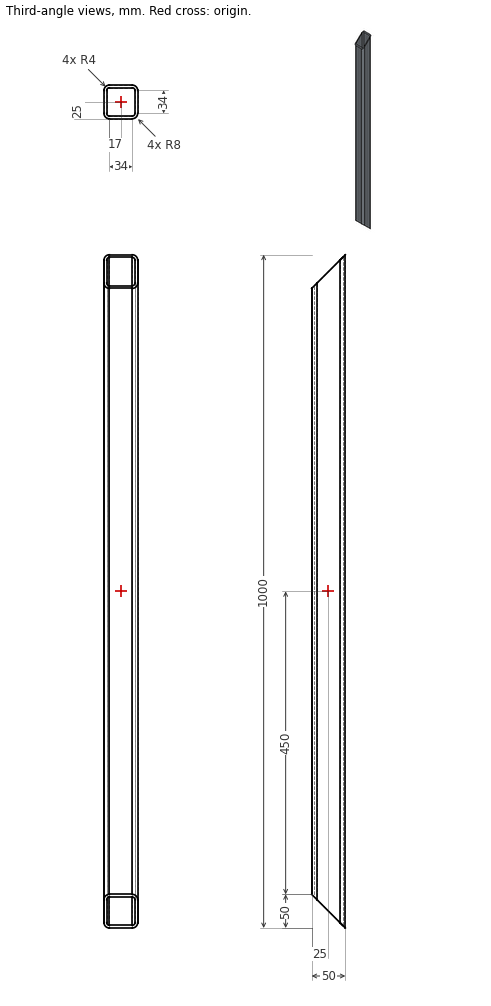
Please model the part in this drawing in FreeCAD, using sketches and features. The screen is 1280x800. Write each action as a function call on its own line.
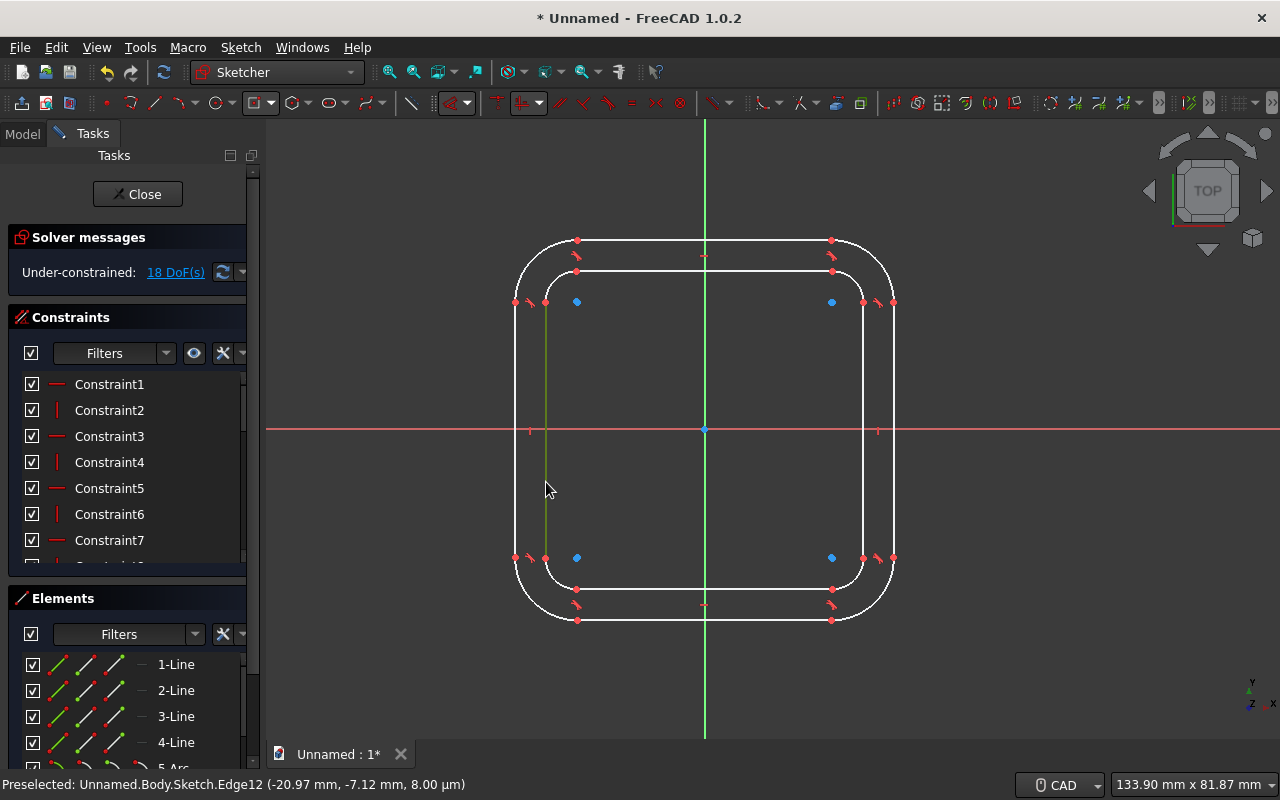
click(549, 572)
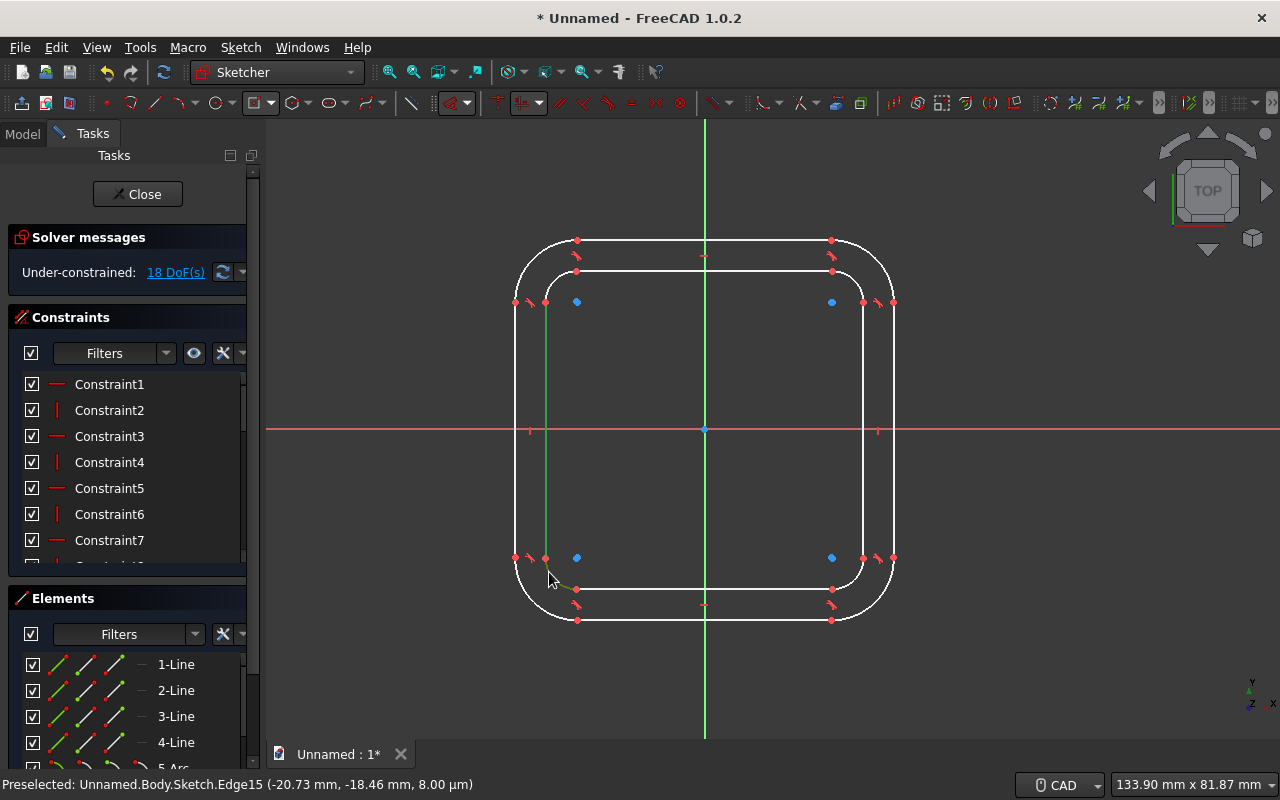
click(608, 104)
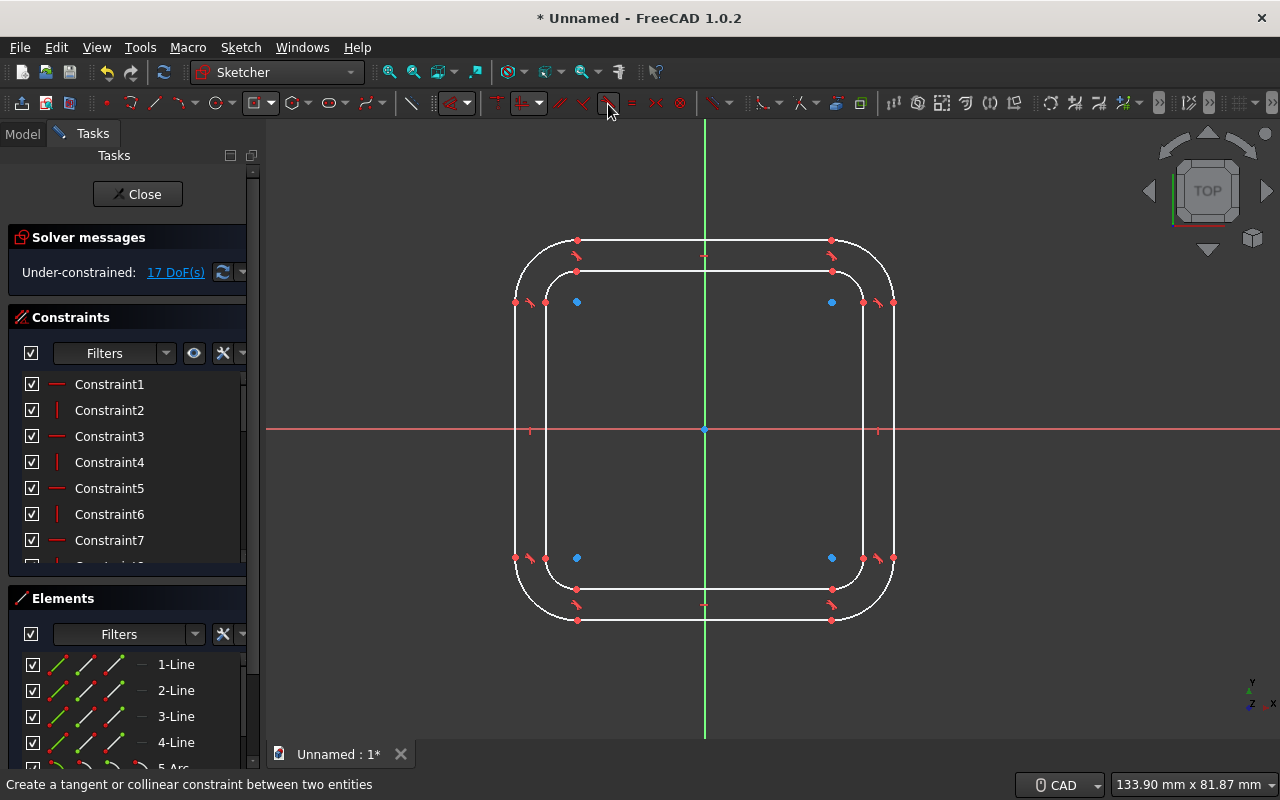
click(546, 482)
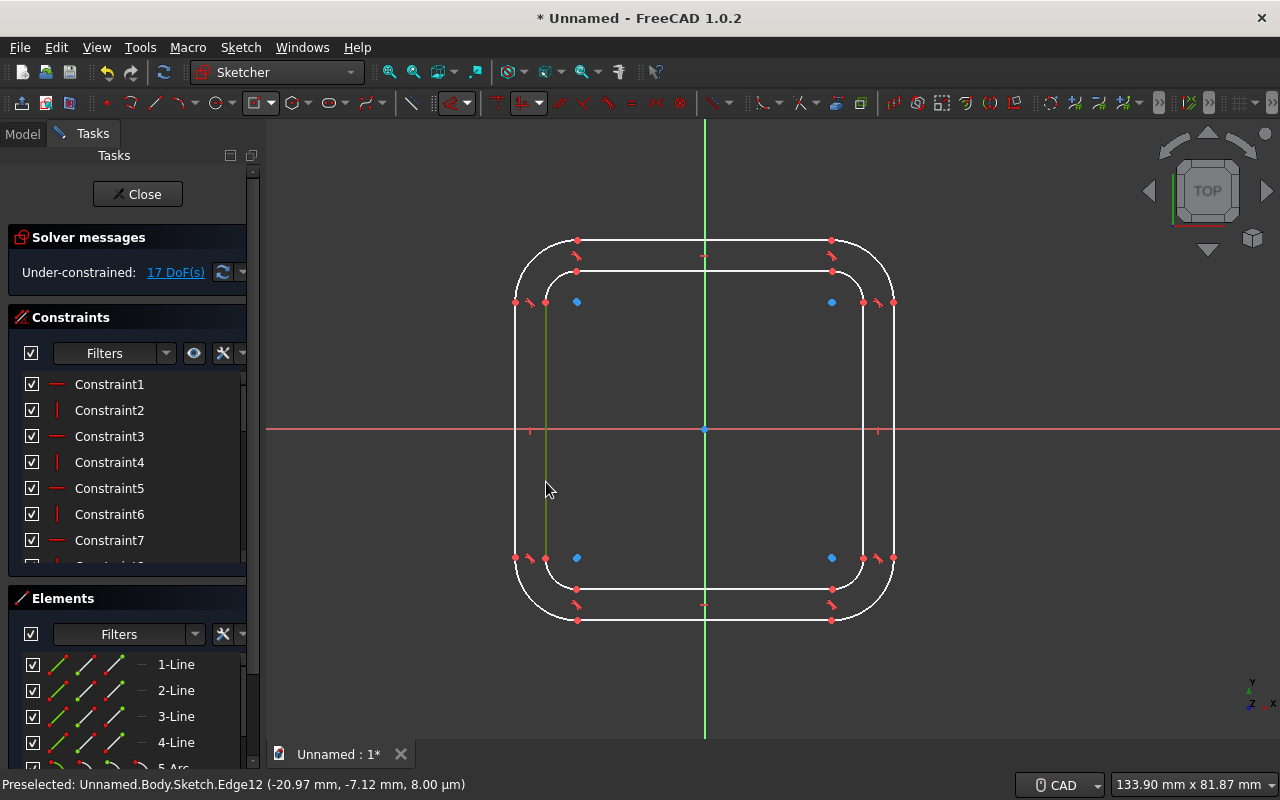
click(562, 275)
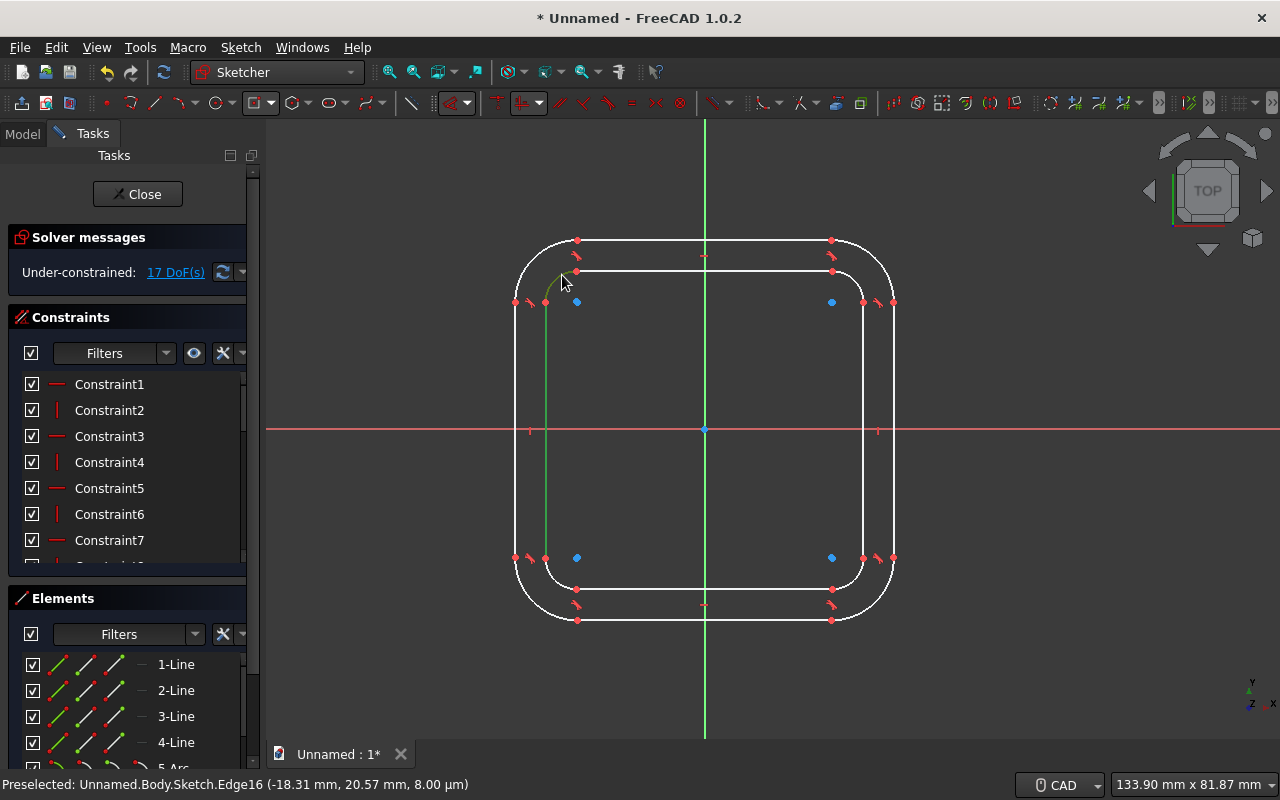
click(608, 104)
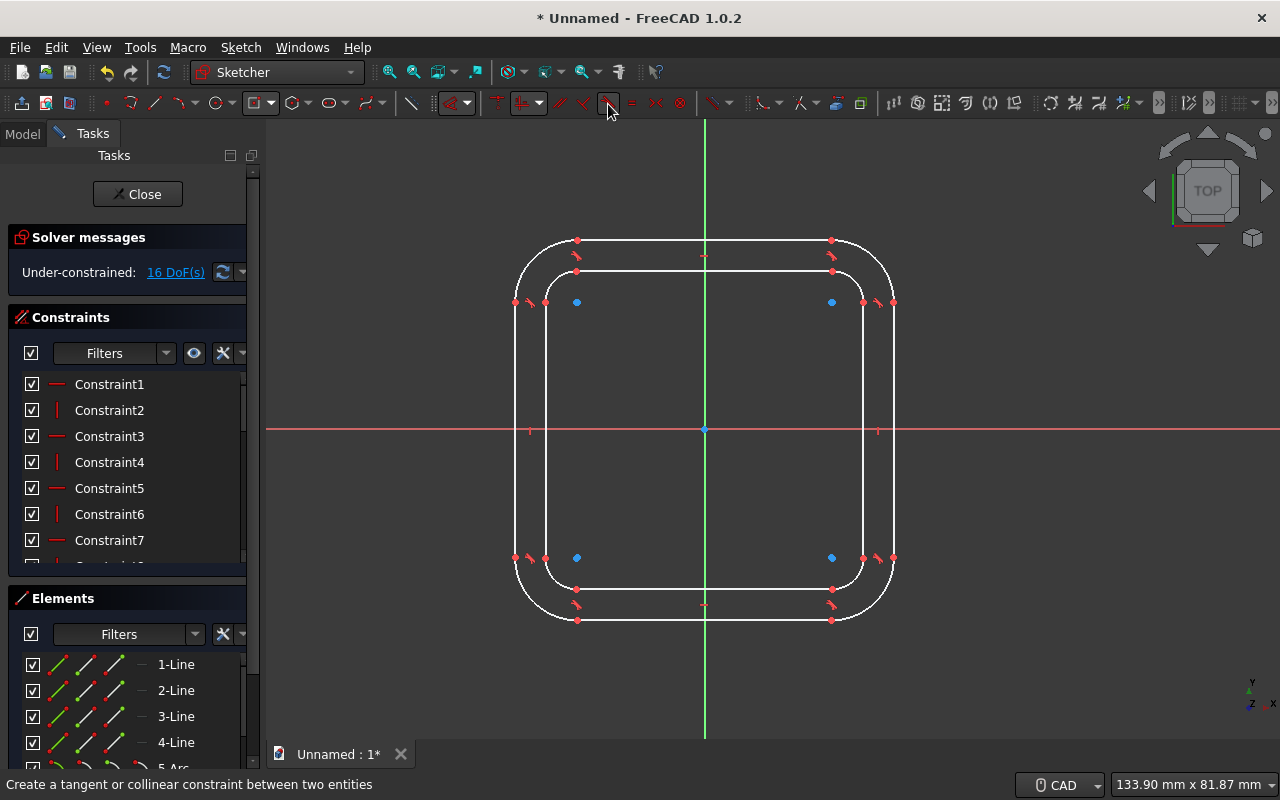
click(887, 274)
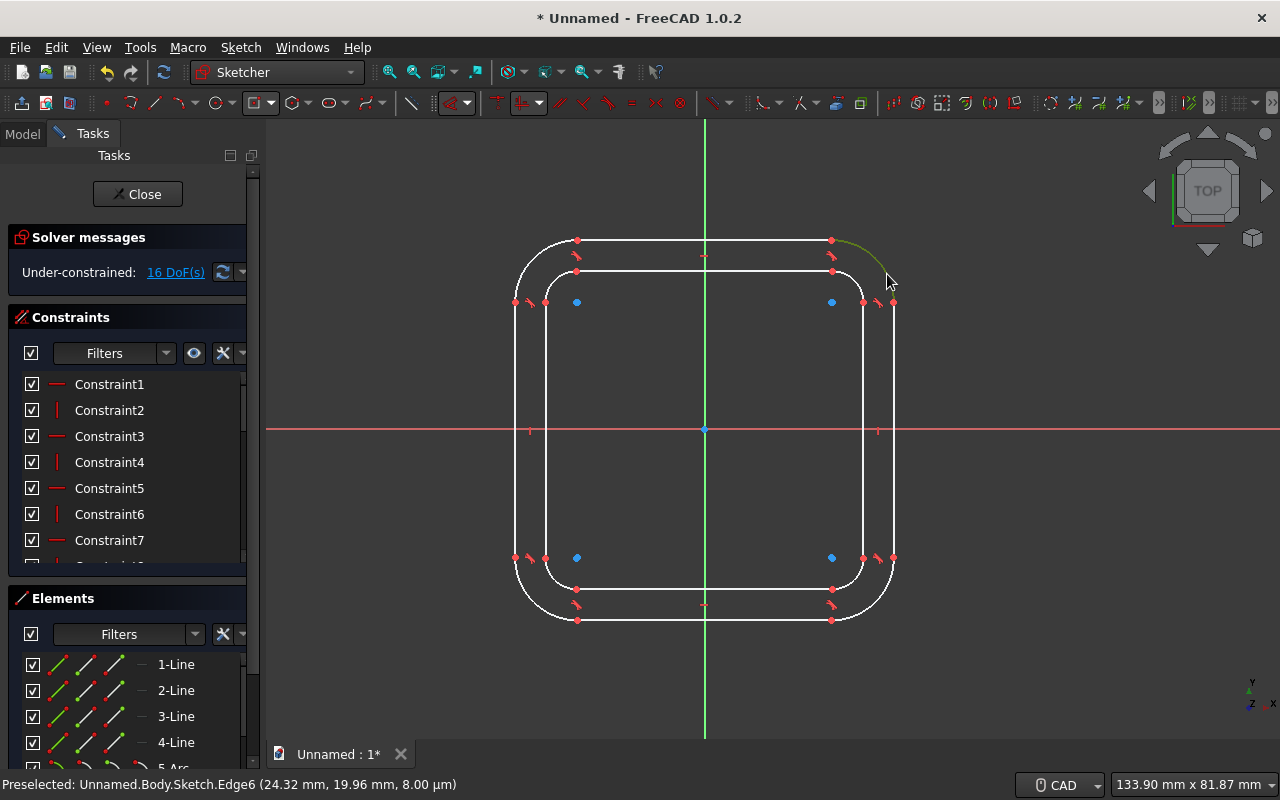
click(860, 288)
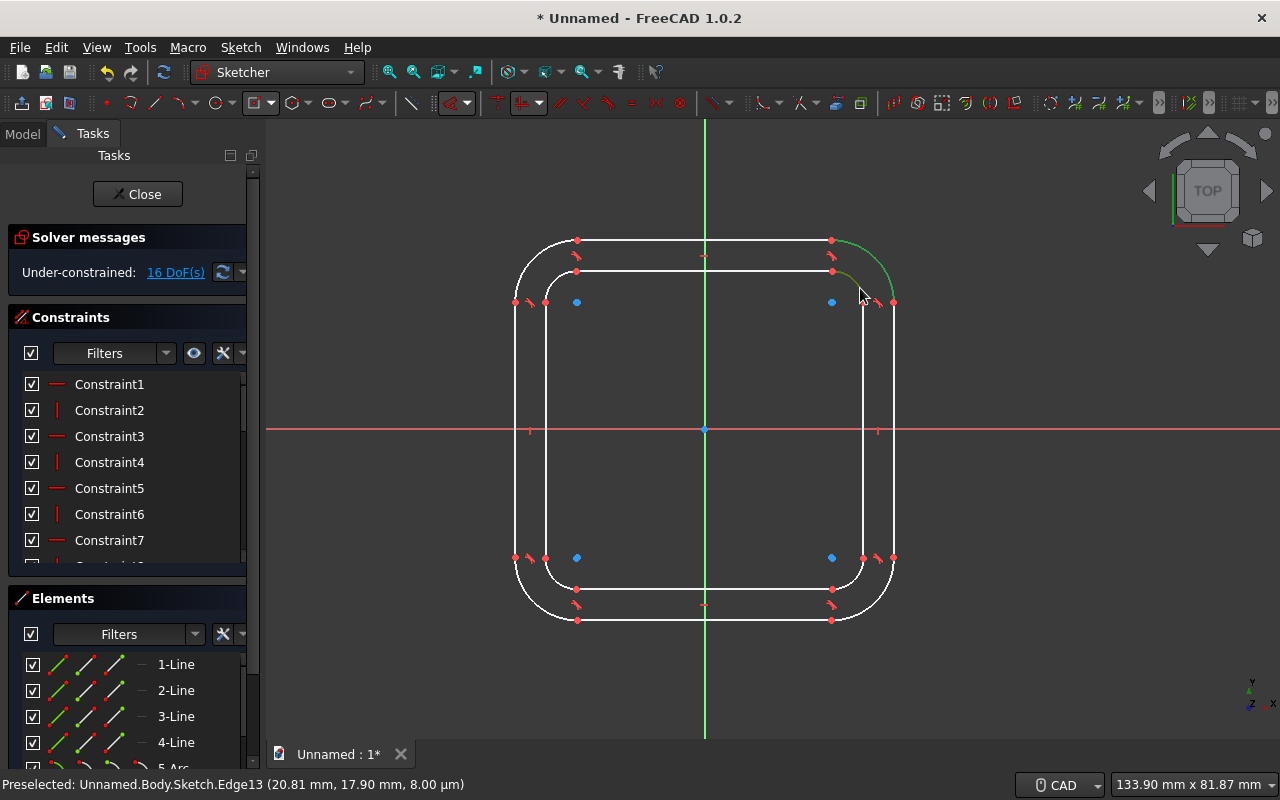
key(c)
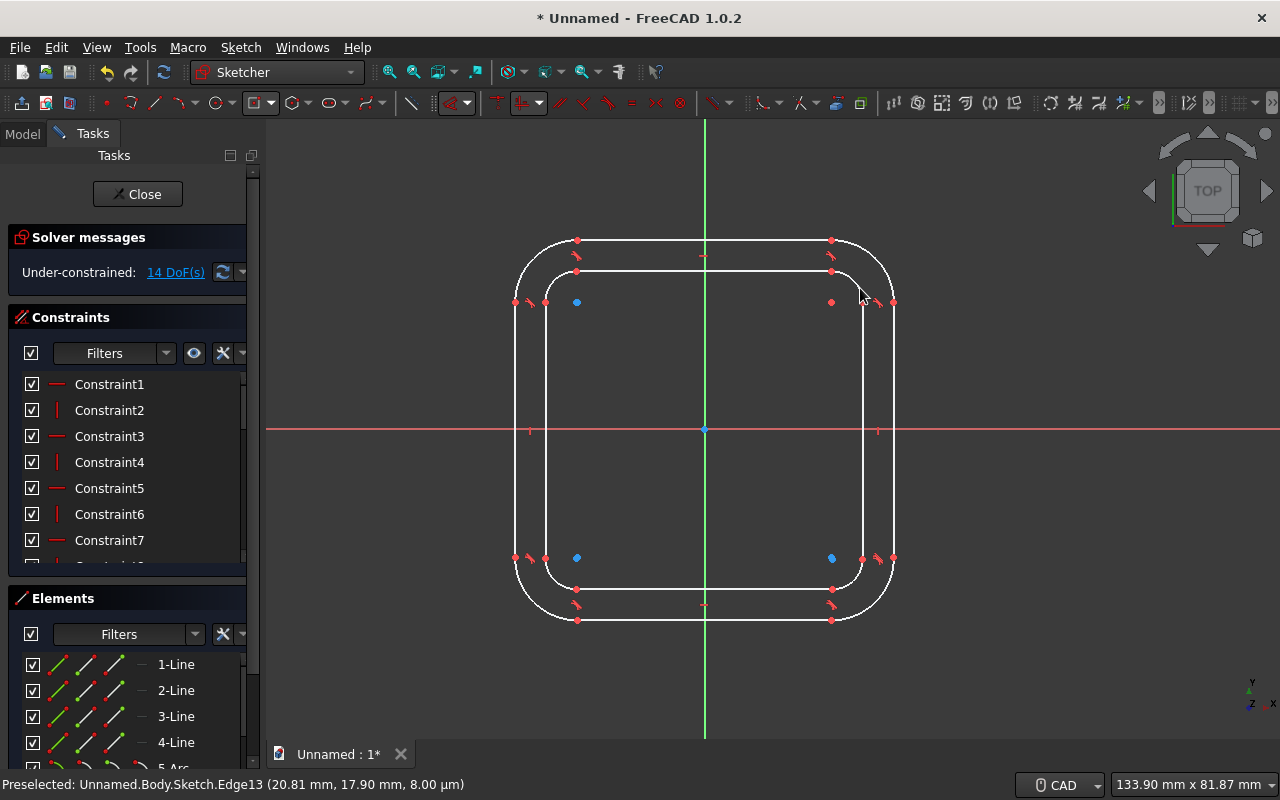
click(860, 614)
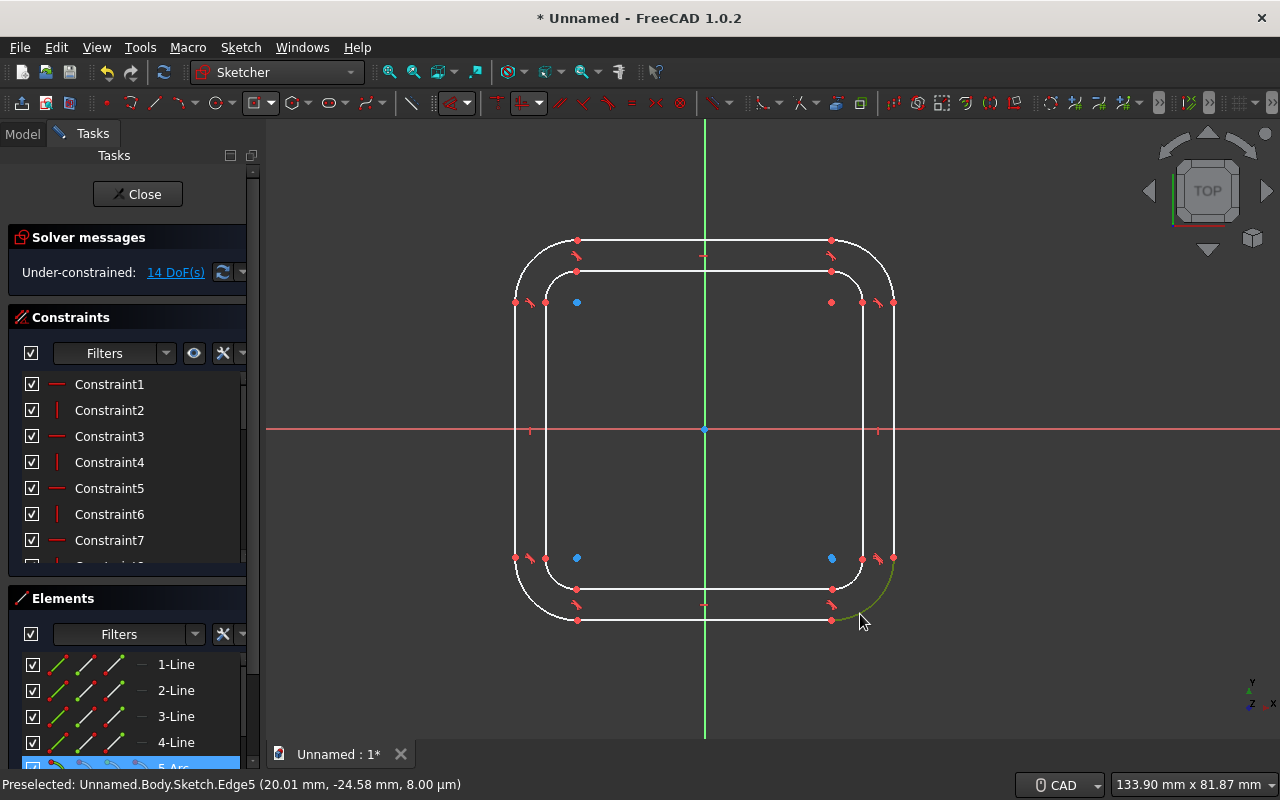
click(846, 586)